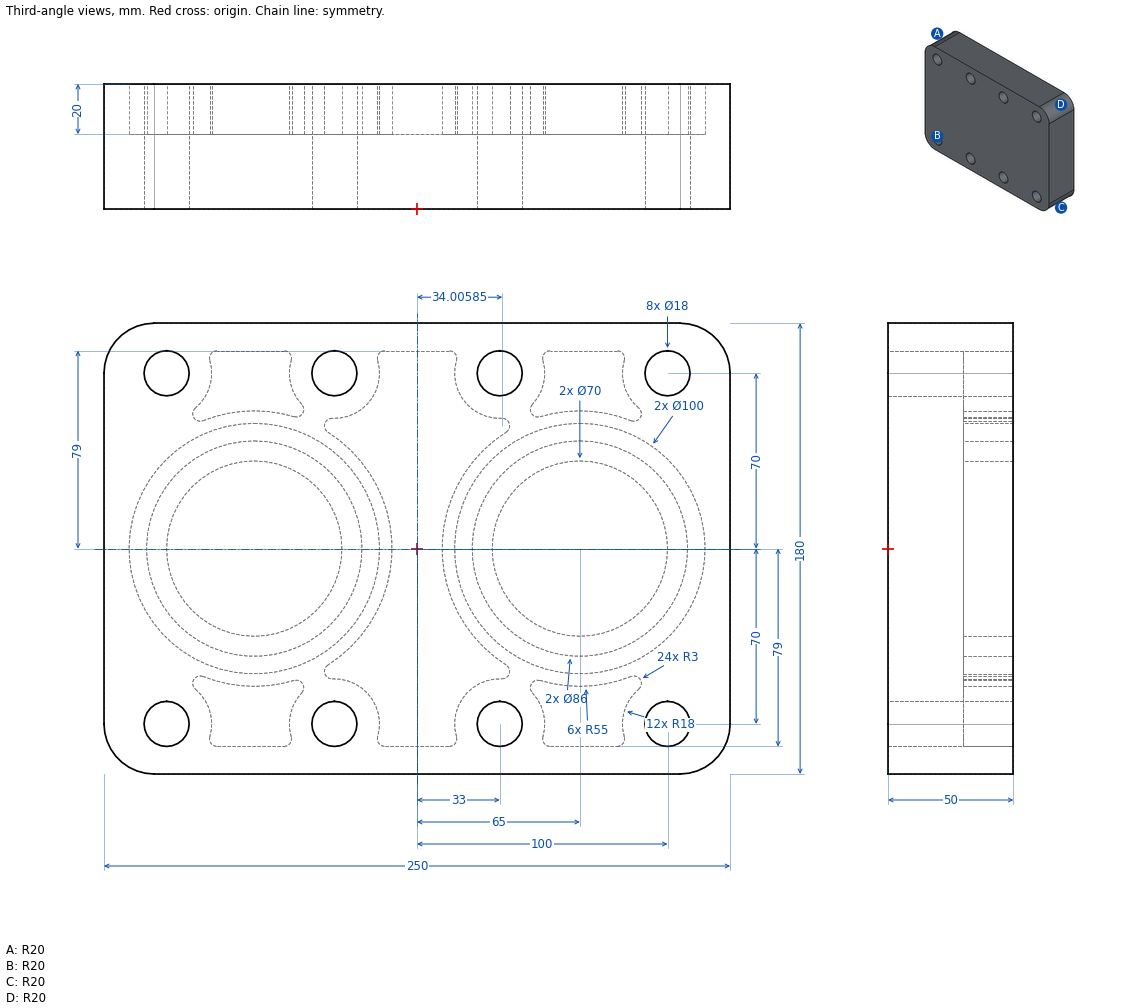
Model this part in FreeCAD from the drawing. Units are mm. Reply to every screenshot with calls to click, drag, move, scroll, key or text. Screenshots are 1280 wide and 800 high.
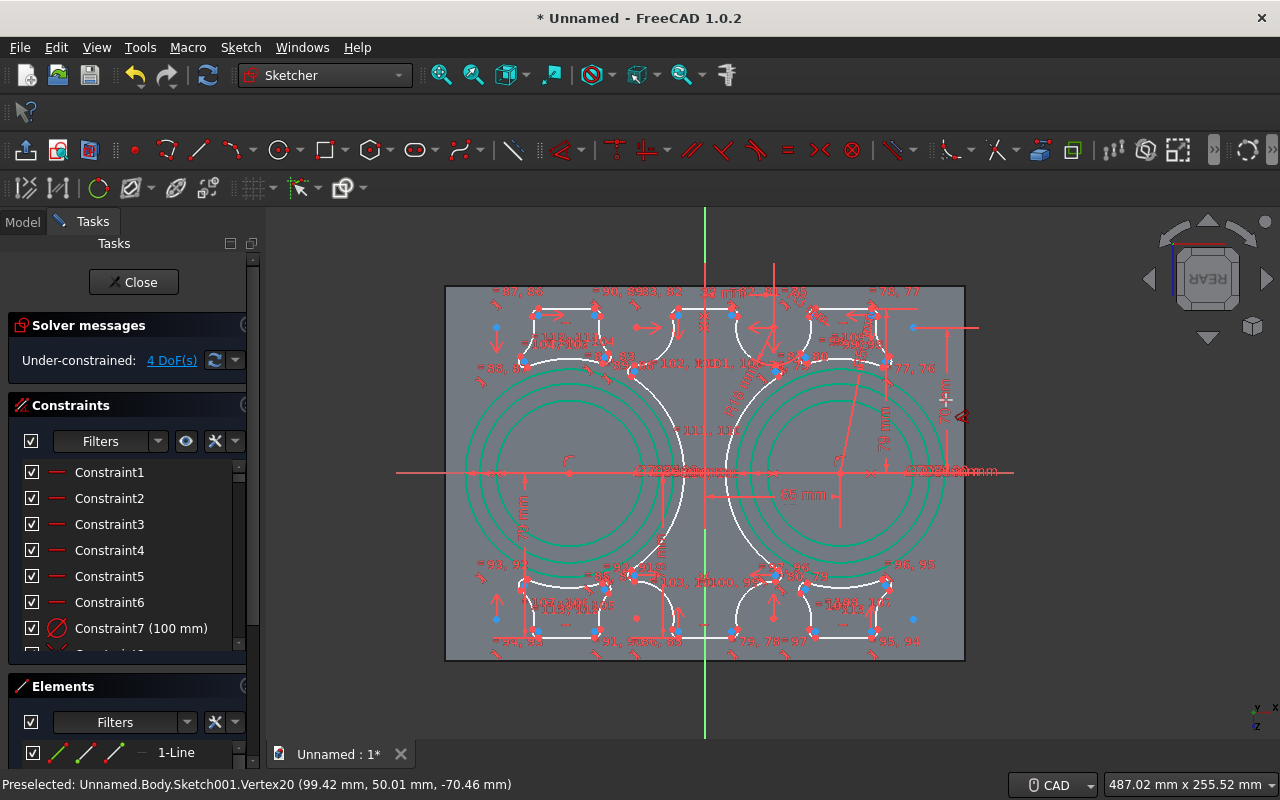
click(497, 328)
click(463, 401)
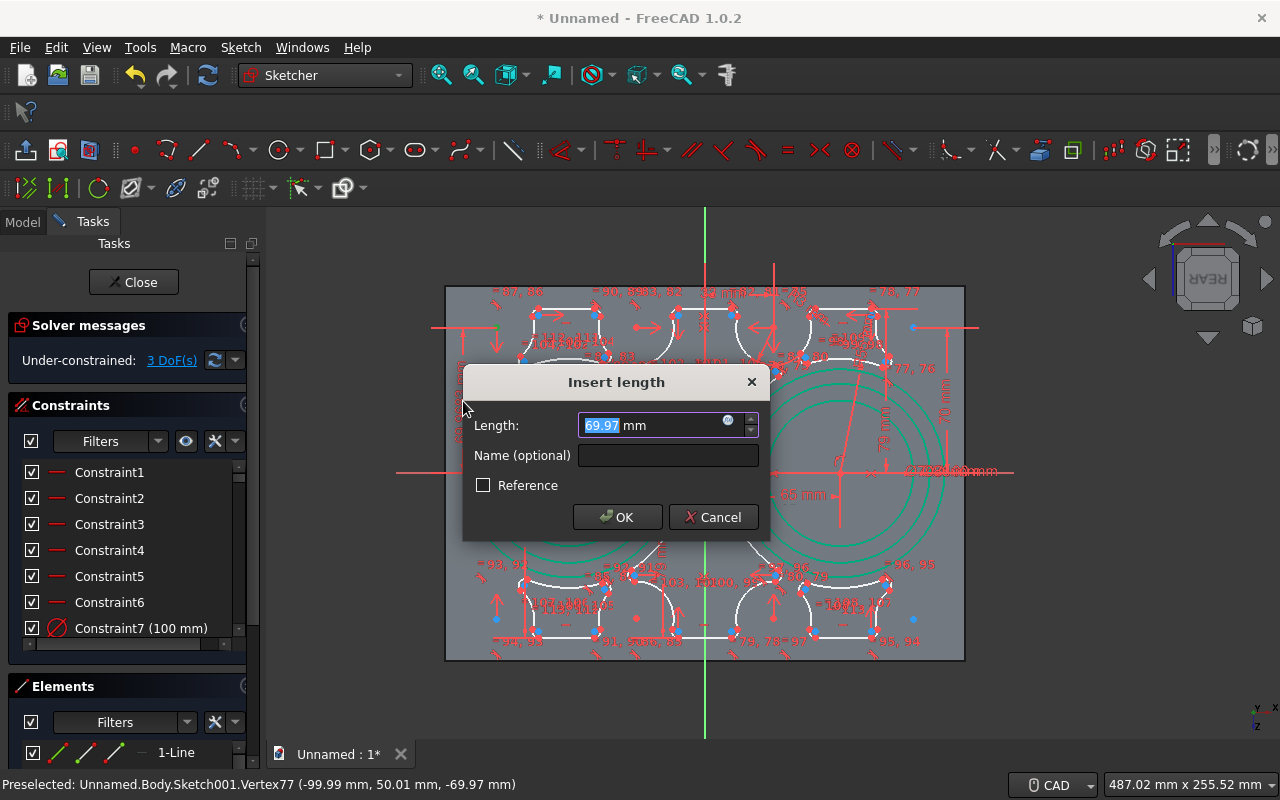
text(70)
key(Return)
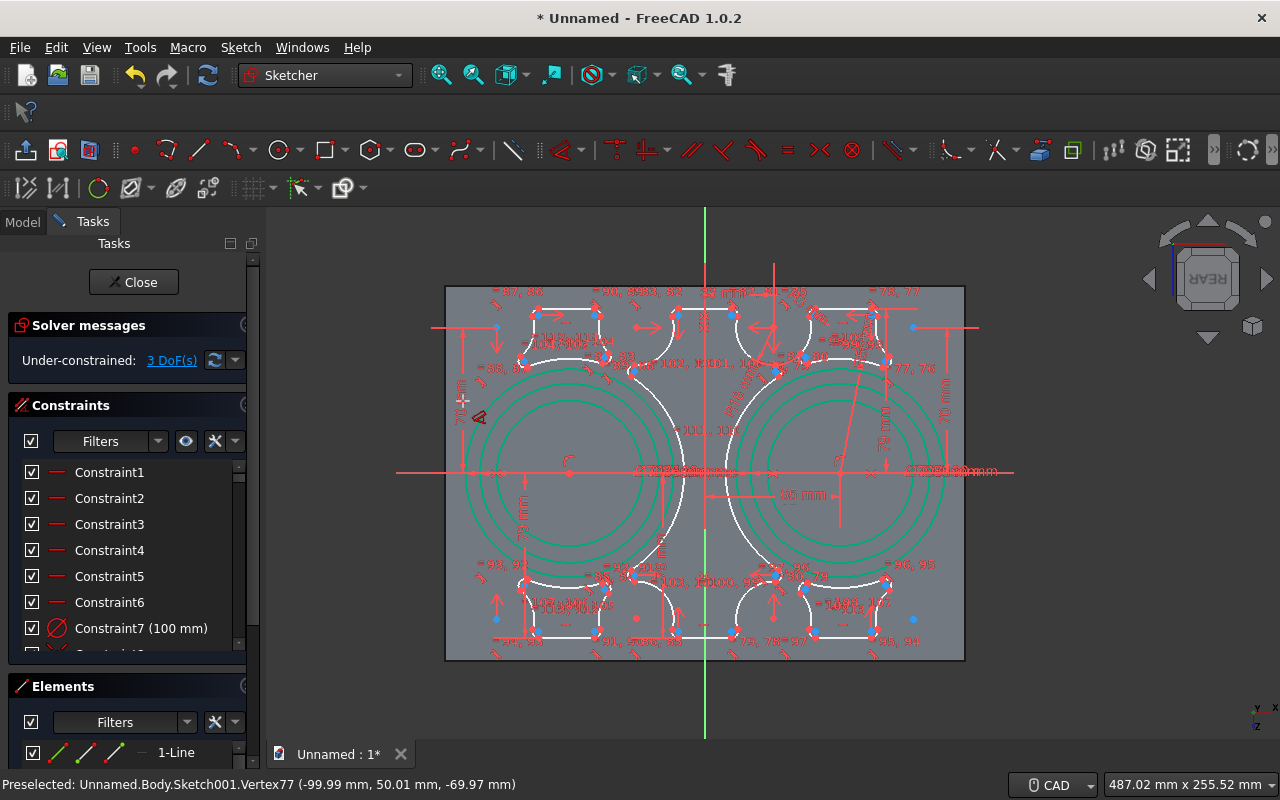
click(913, 619)
click(947, 546)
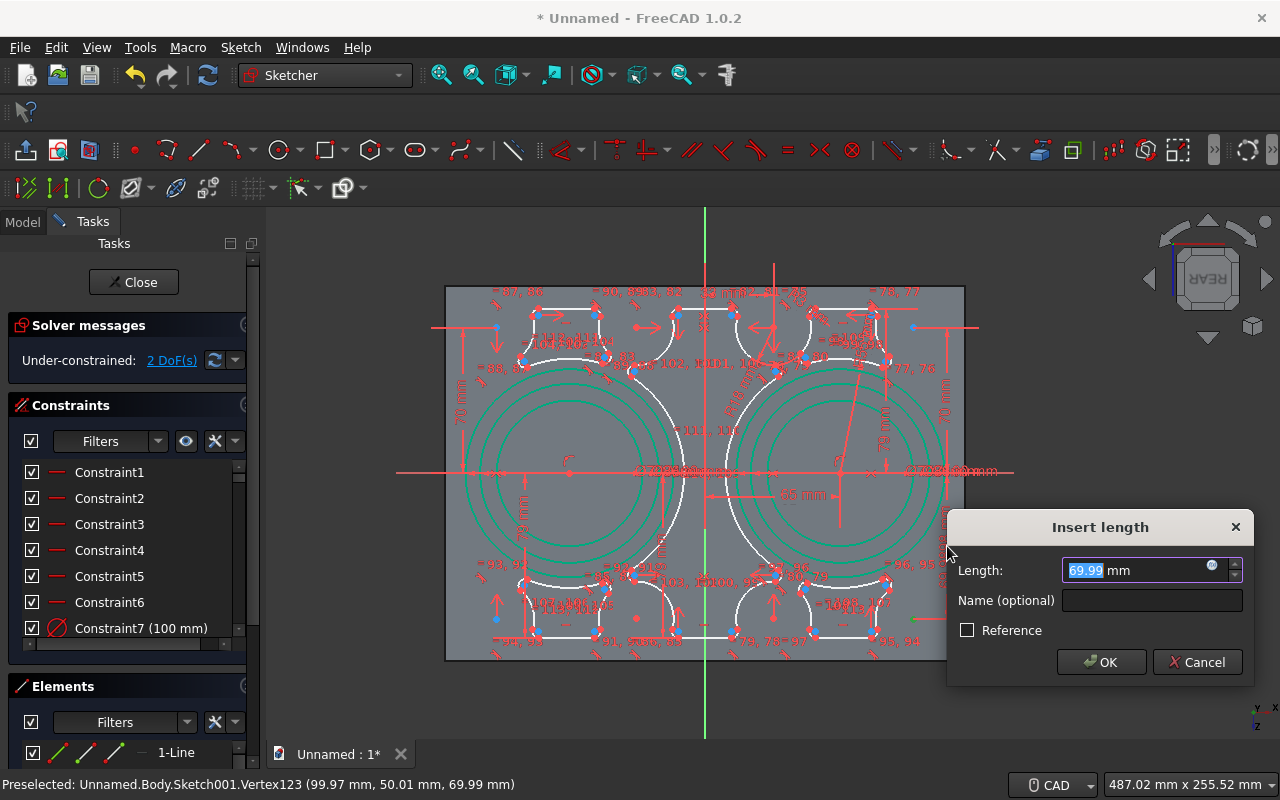
text(70)
key(Return)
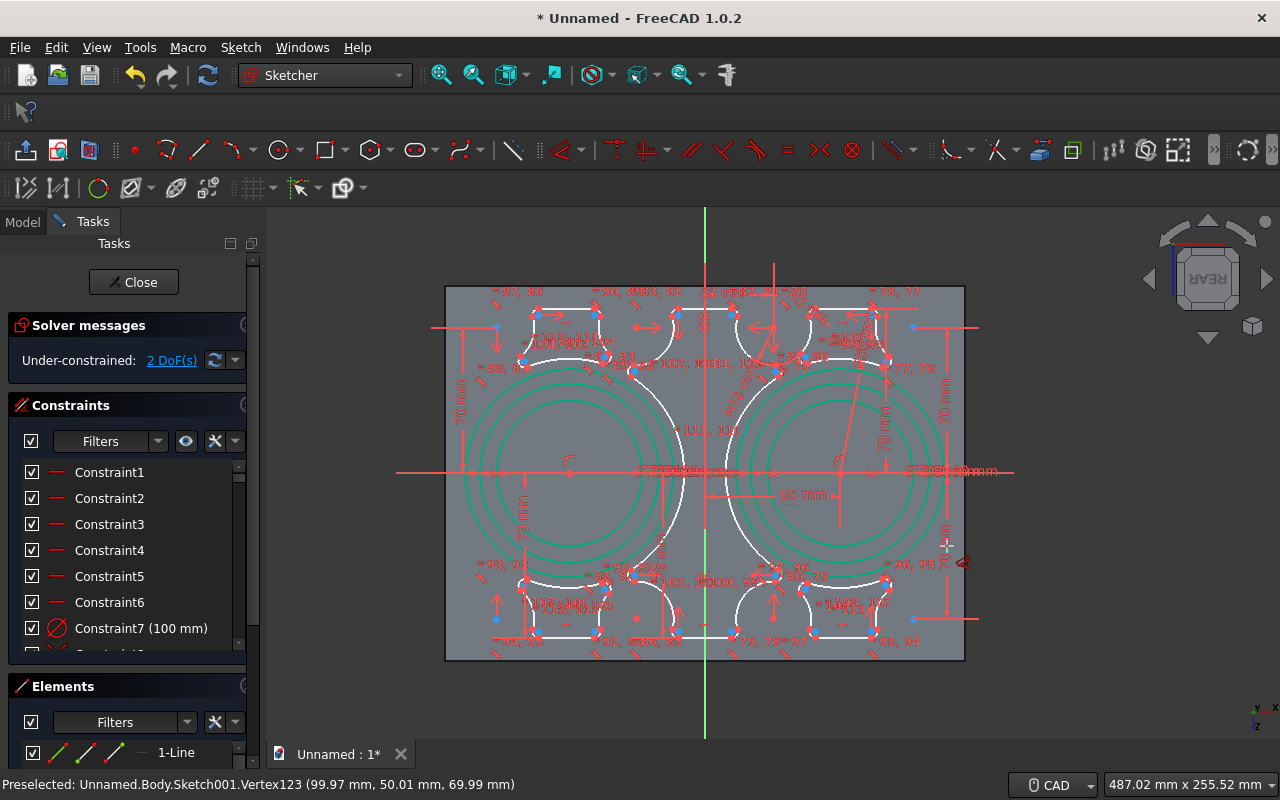
click(913, 328)
click(882, 294)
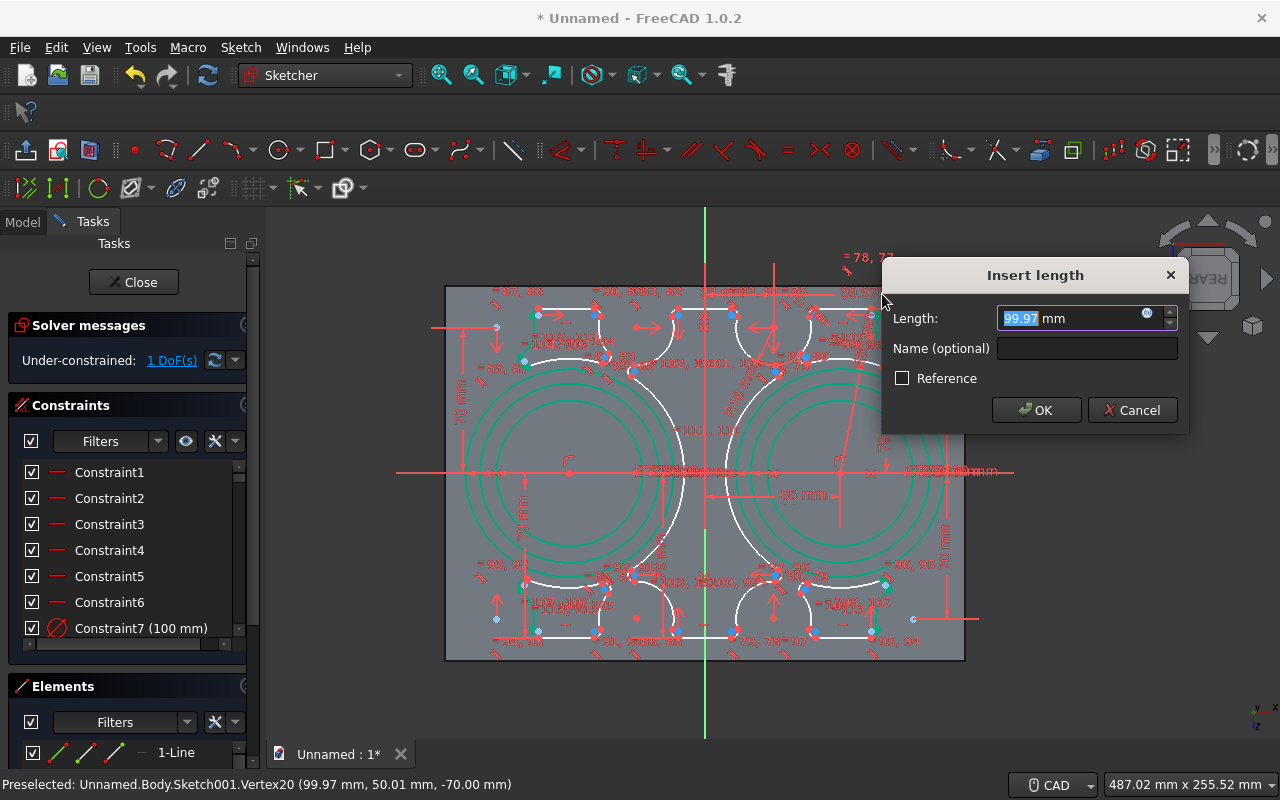
text(100)
key(Return)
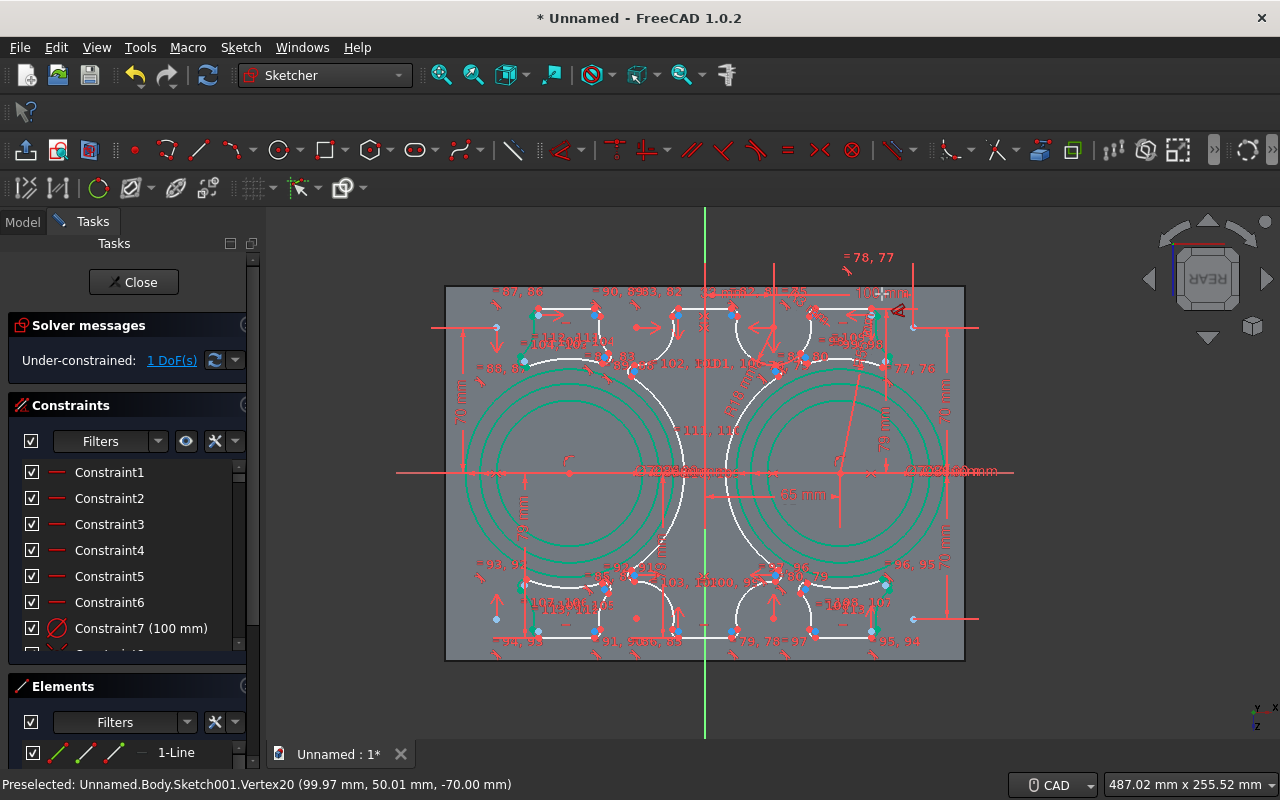
scroll(775, 575, up, 4)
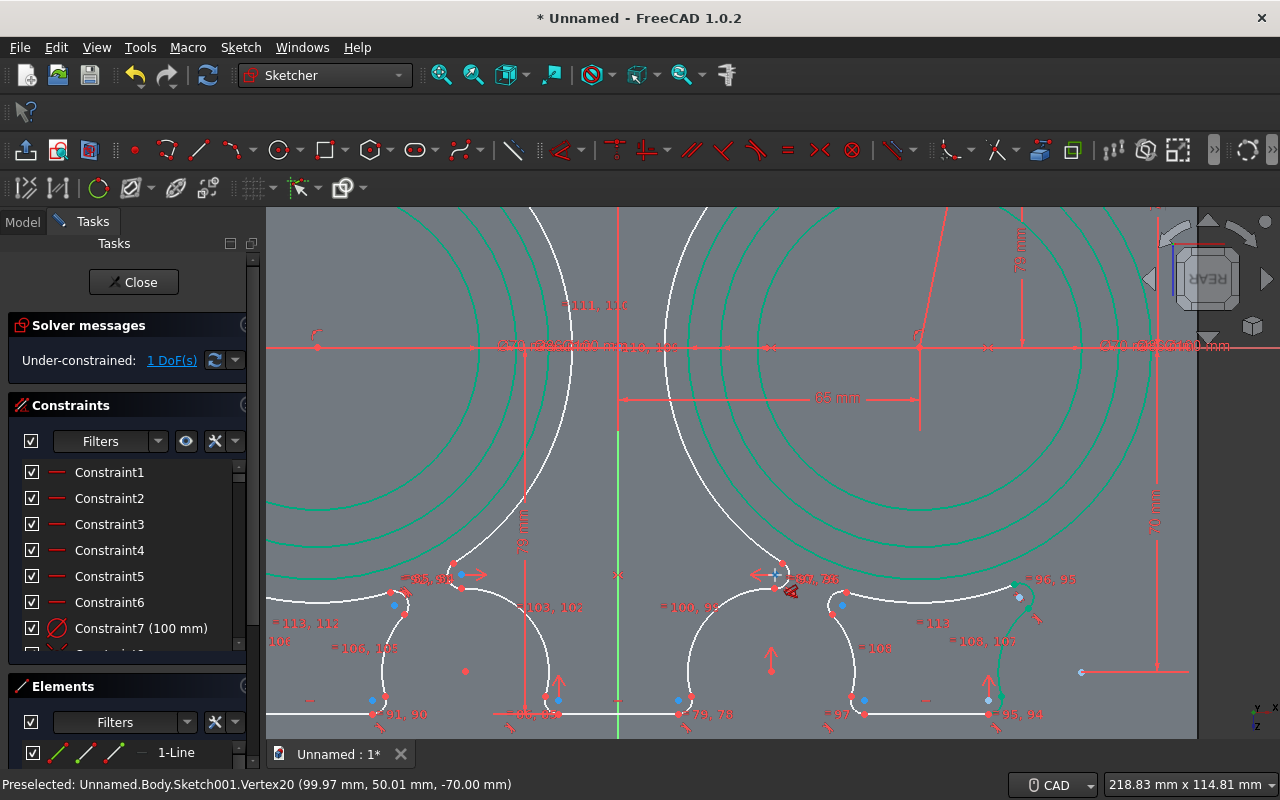
click(775, 575)
click(697, 609)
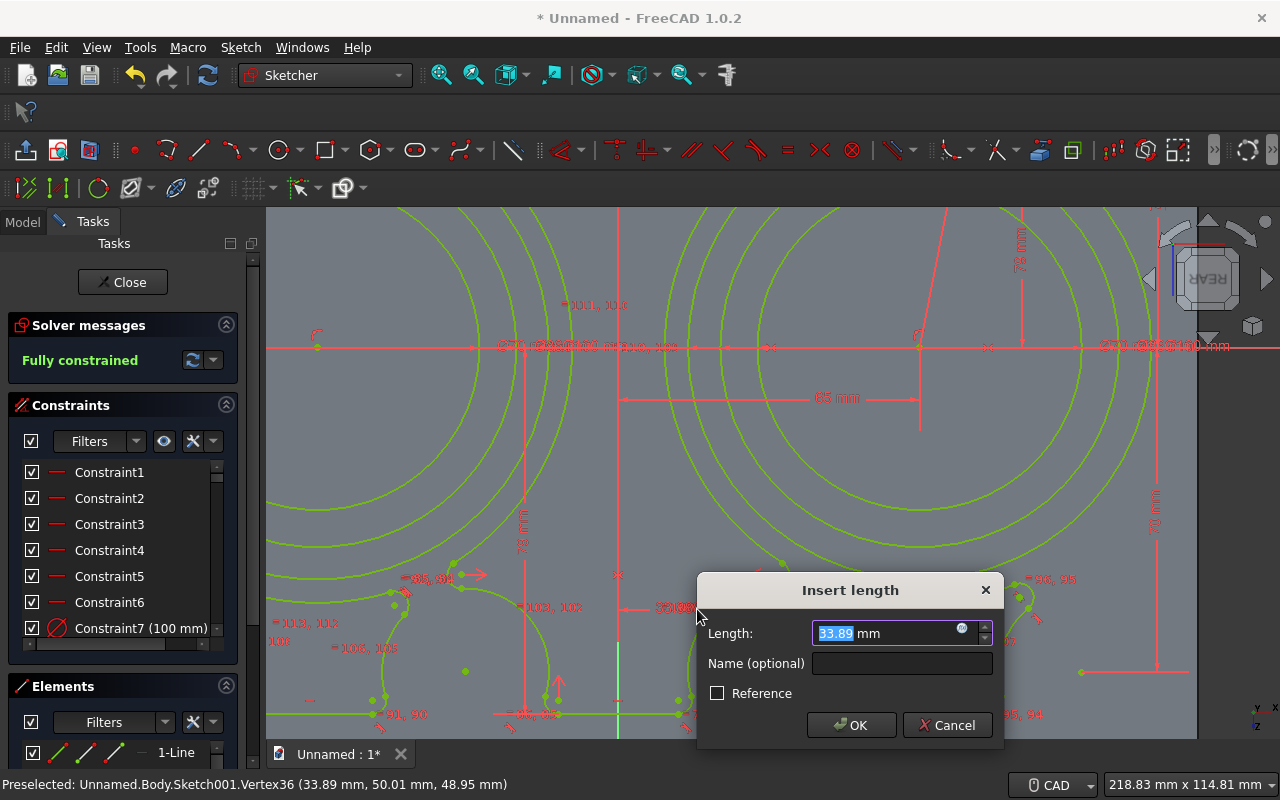
text(34.00585)
key(Return)
key(Escape)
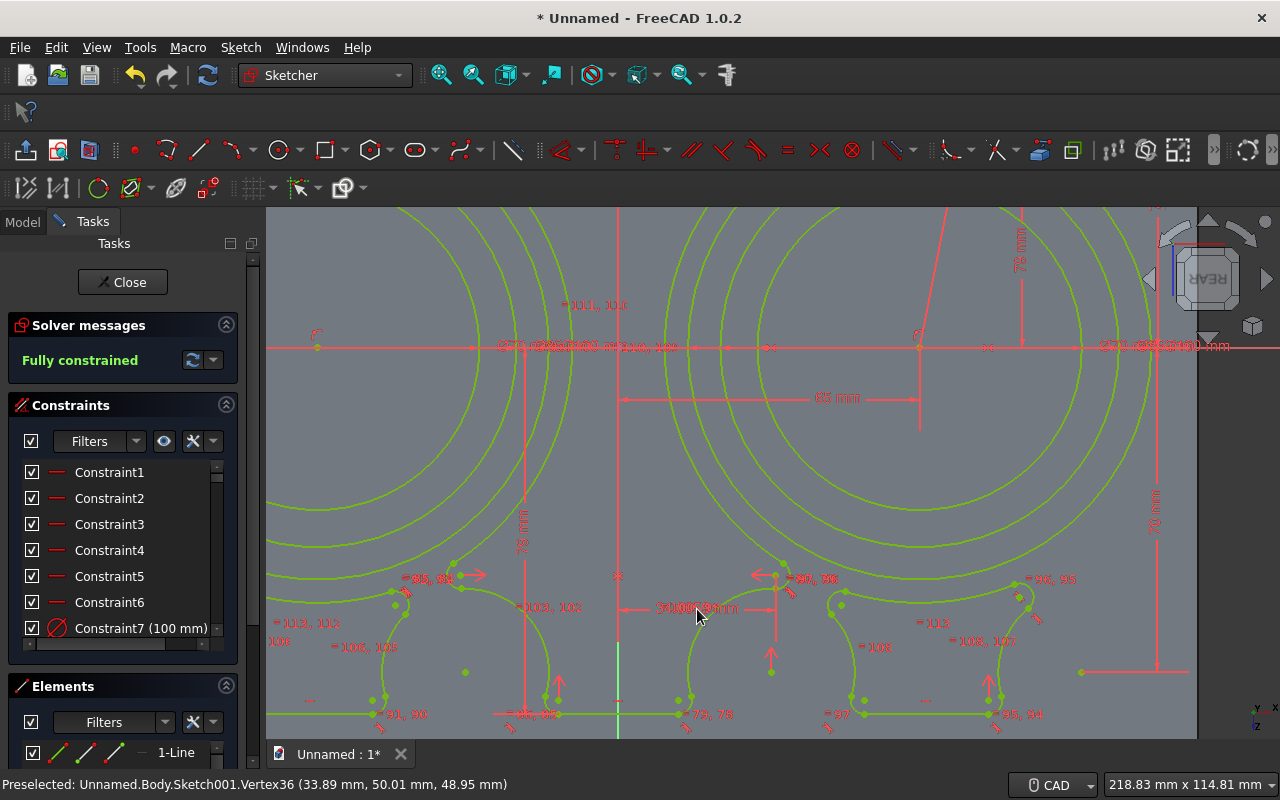
click(123, 282)